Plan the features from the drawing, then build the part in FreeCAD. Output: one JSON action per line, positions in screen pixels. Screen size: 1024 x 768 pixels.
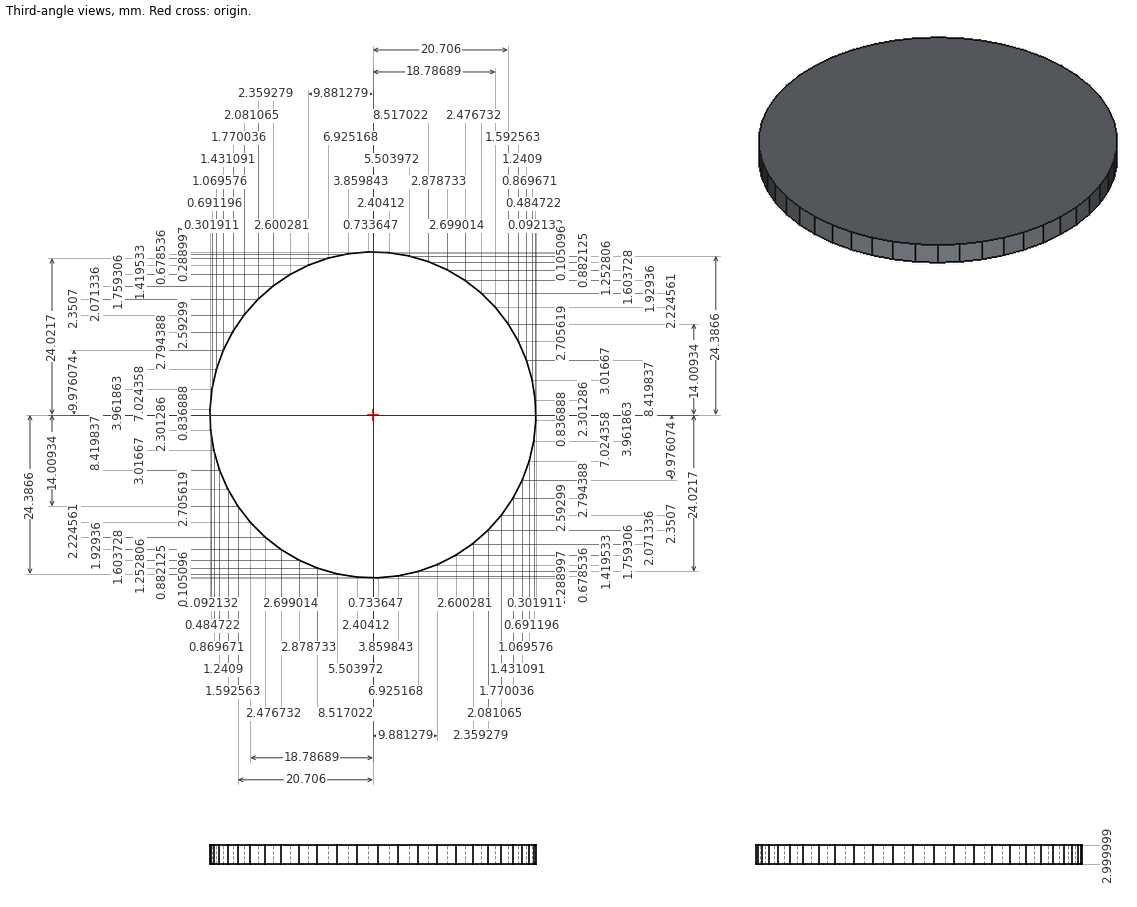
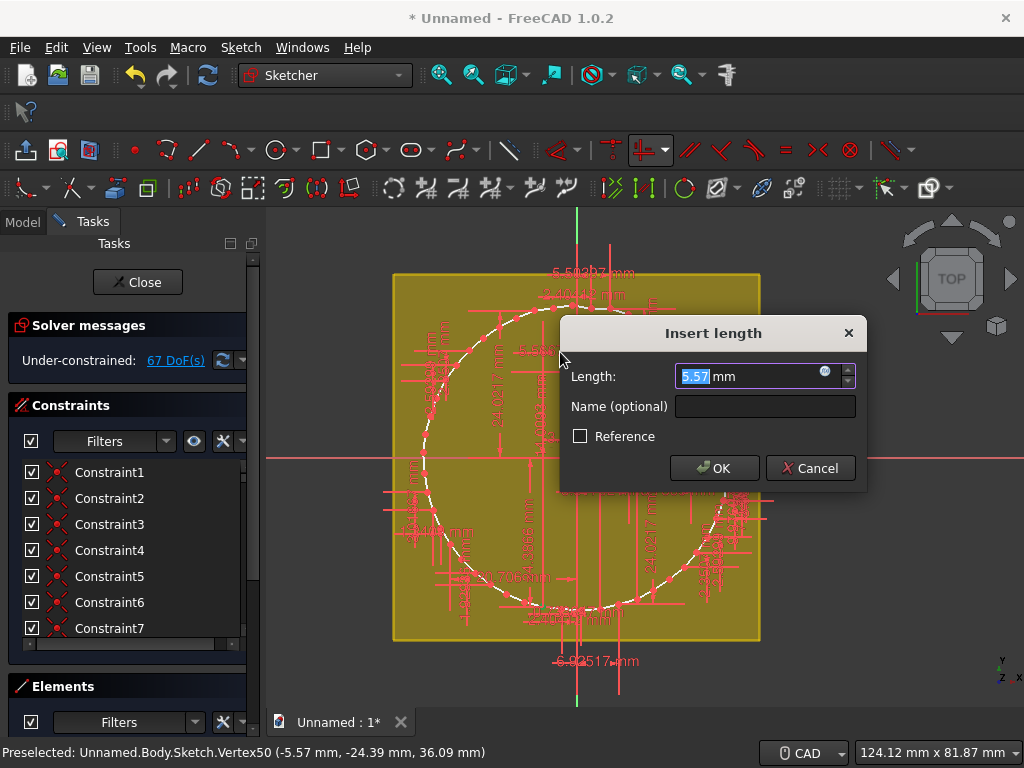
{"action": "type", "text": "5.503972"}
{"action": "key", "text": "Return"}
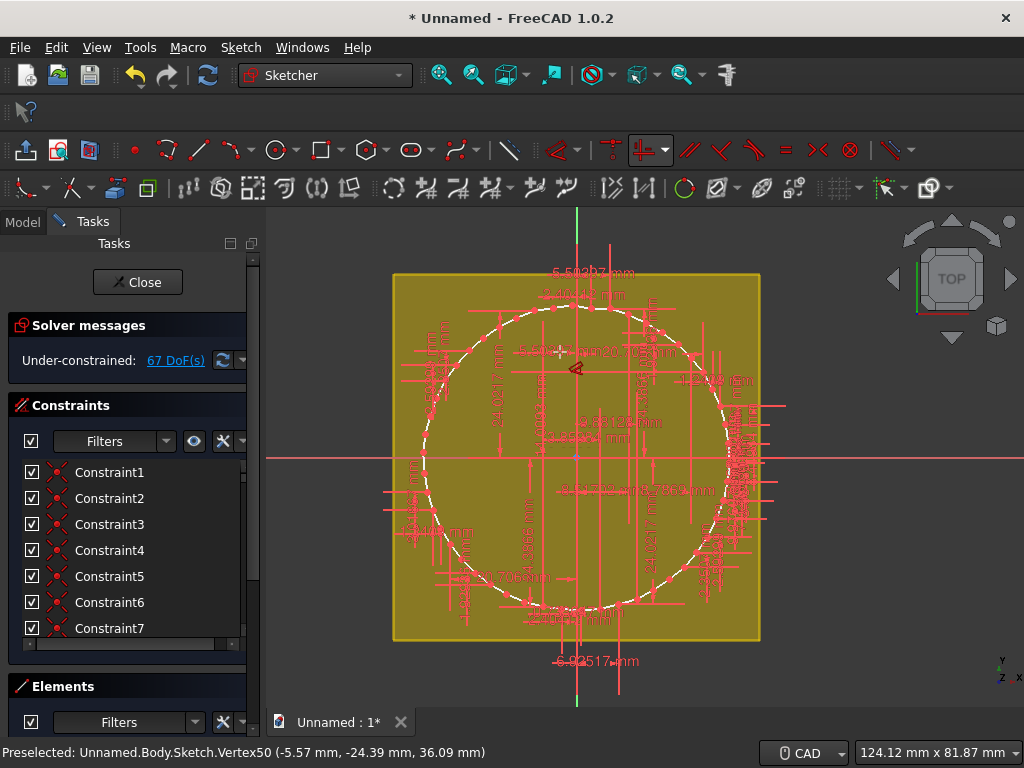
{"action": "left_click", "coordinate": [525, 602]}
{"action": "left_click", "coordinate": [551, 328]}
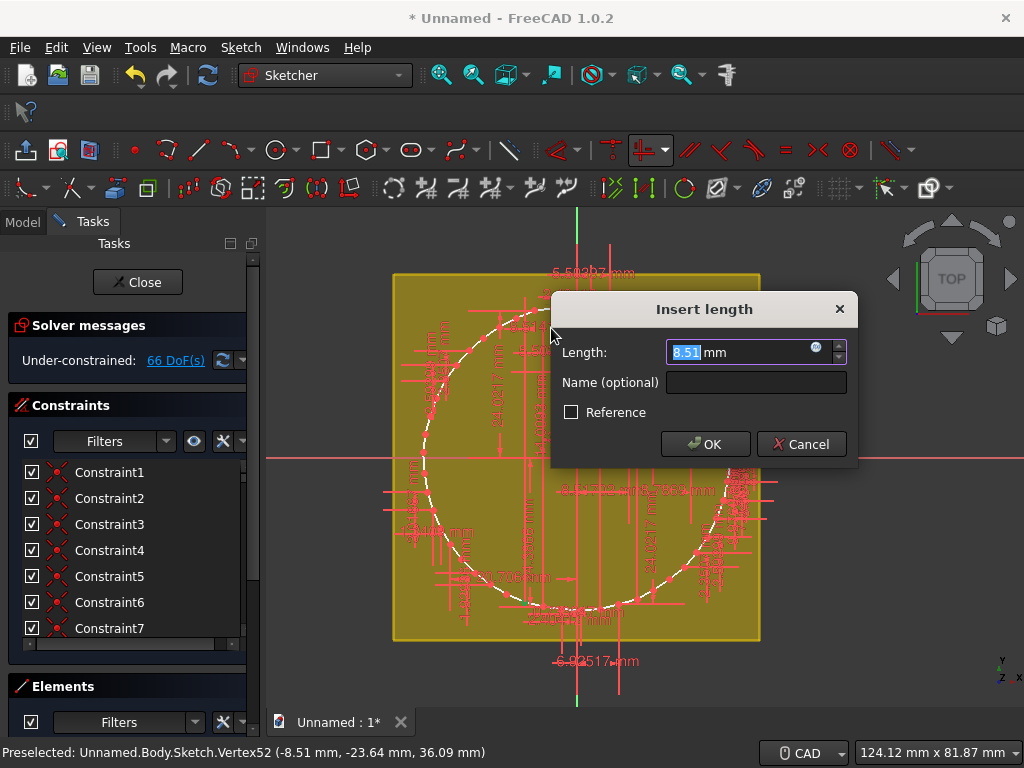
{"action": "type", "text": "8.517022"}
{"action": "key", "text": "Return"}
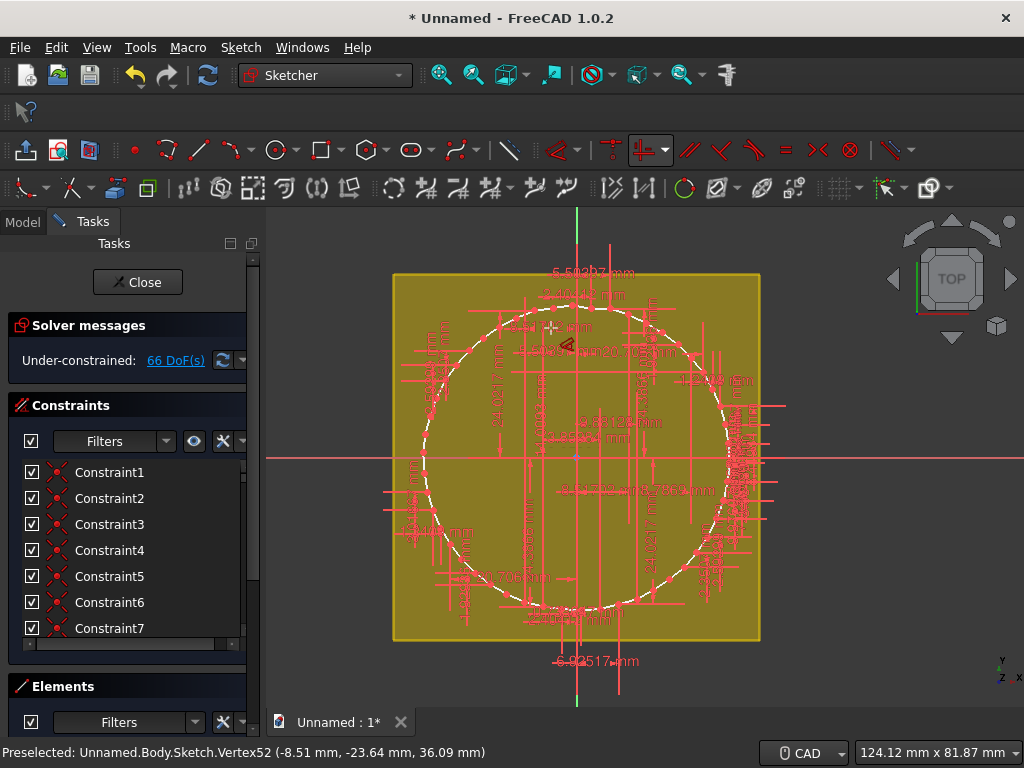
{"action": "left_click", "coordinate": [462, 559]}
{"action": "left_click", "coordinate": [493, 617]}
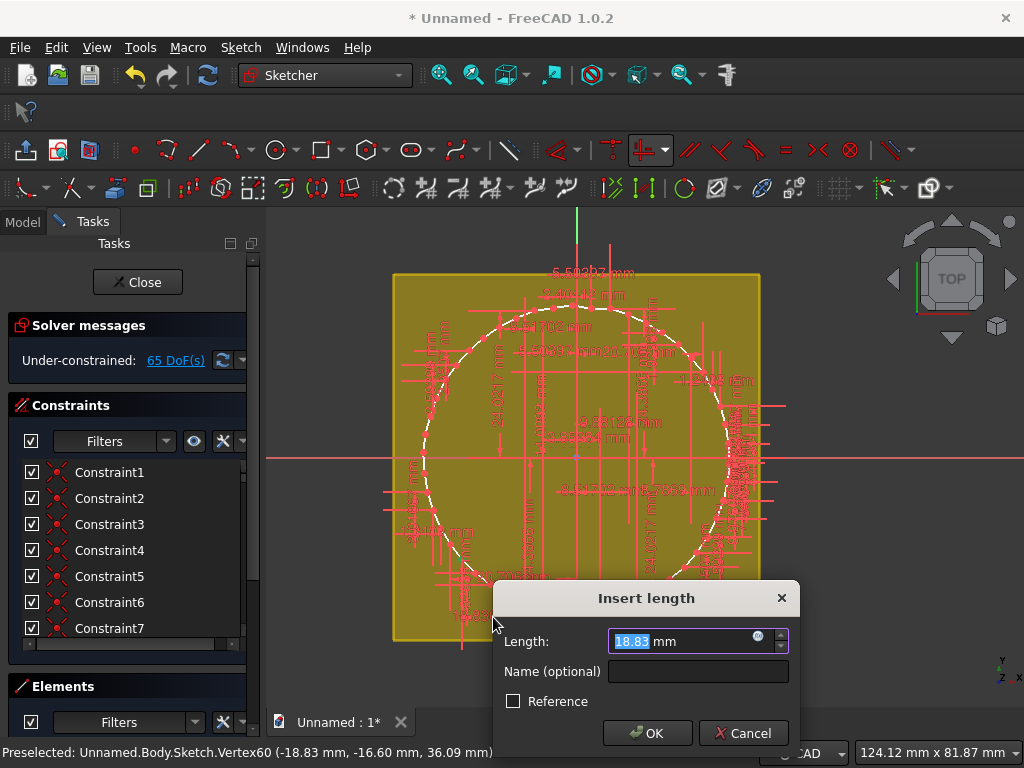
{"action": "type", "text": "18.78689"}
{"action": "key", "text": "Return"}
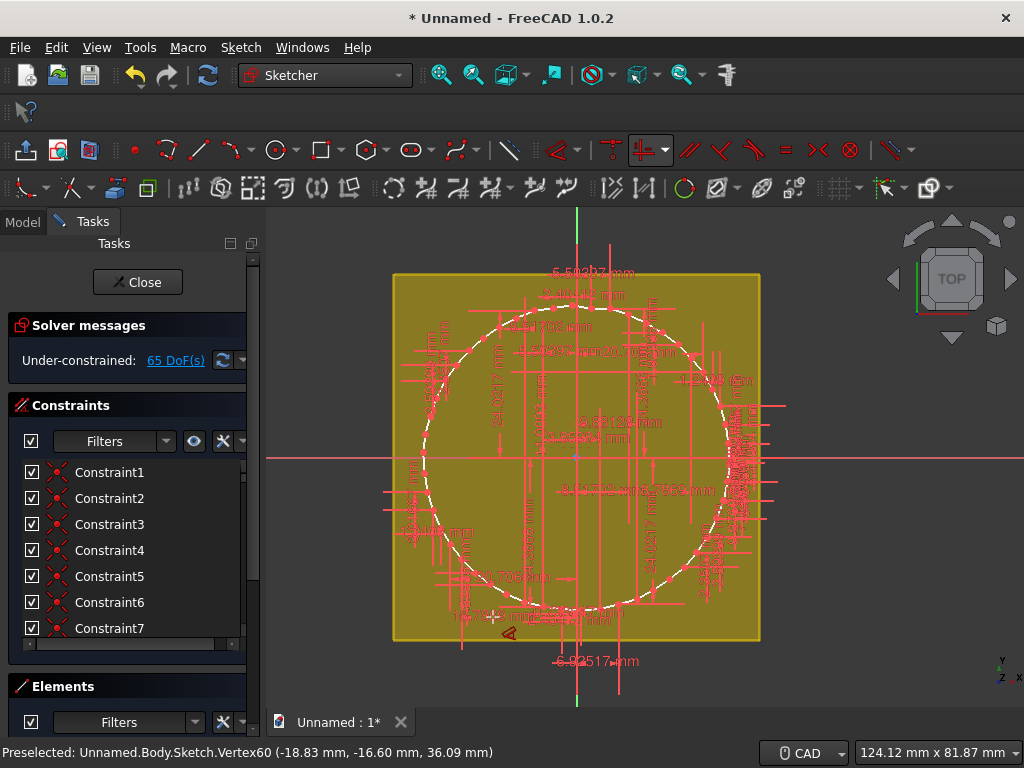
{"action": "left_click", "coordinate": [450, 544]}
{"action": "left_click", "coordinate": [392, 481]}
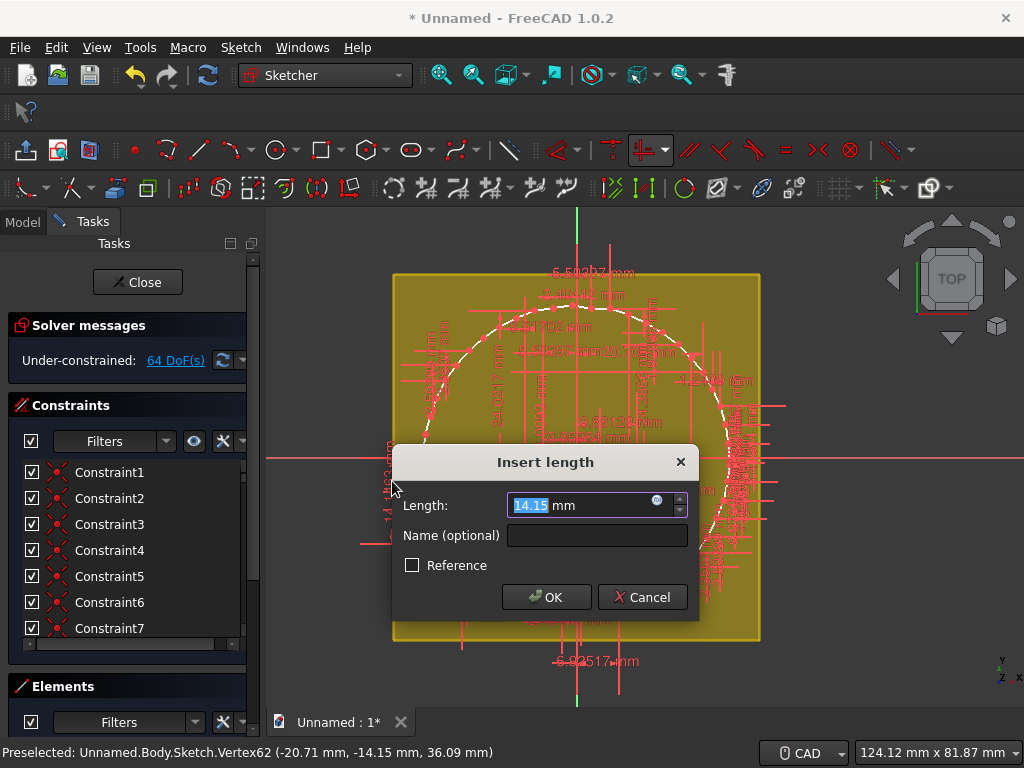
{"action": "type", "text": "14.00934"}
{"action": "key", "text": "Return"}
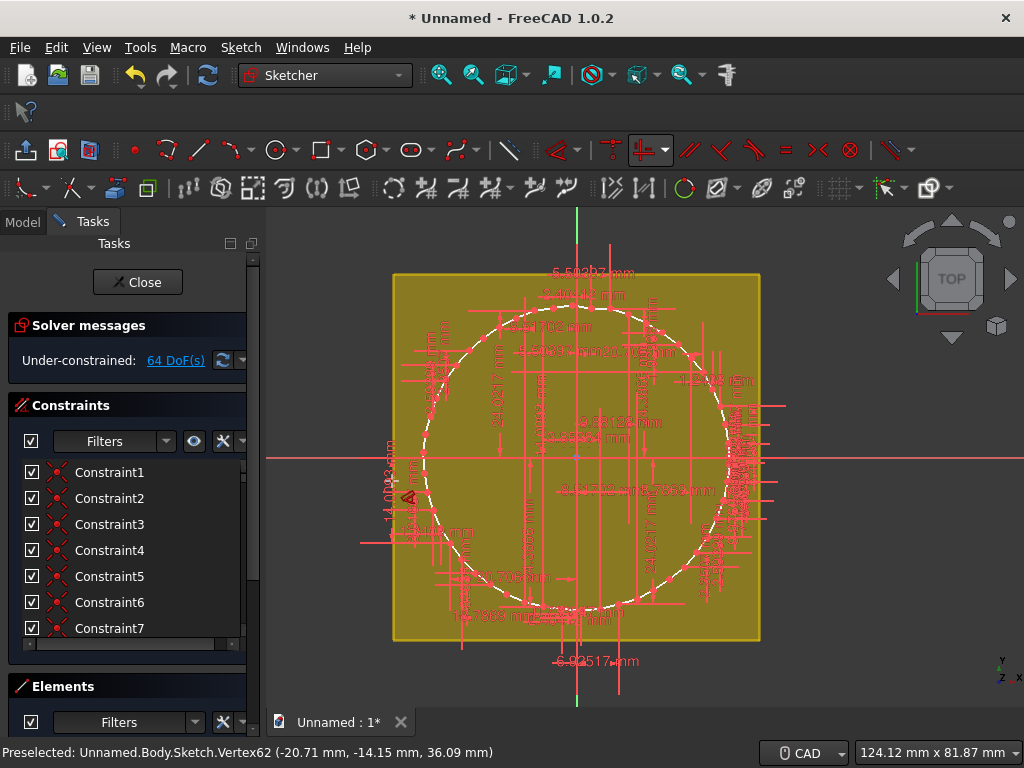
{"action": "left_click", "coordinate": [433, 510]}
{"action": "left_click", "coordinate": [327, 503]}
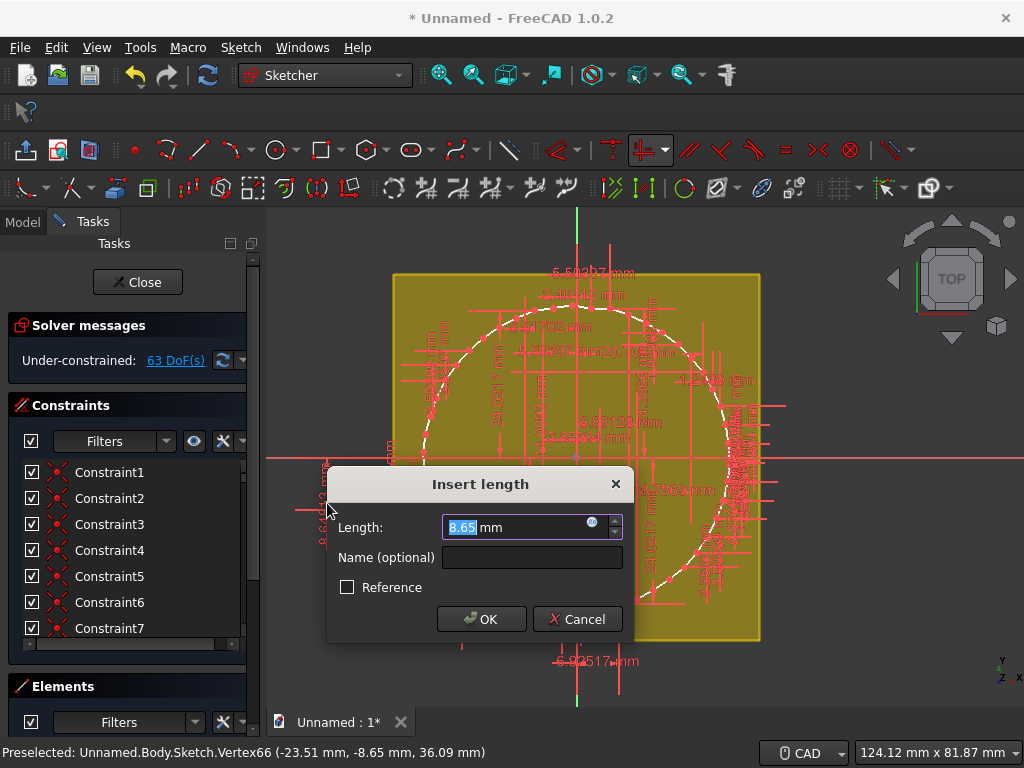
{"action": "type", "text": "8.419837"}
{"action": "key", "text": "Return"}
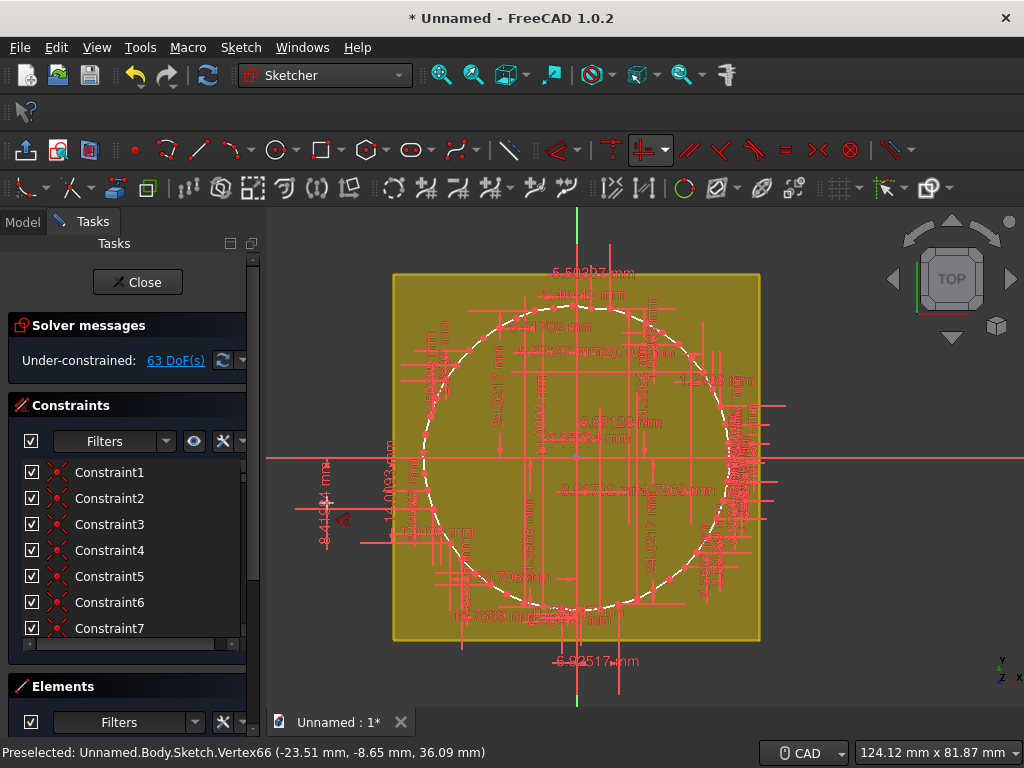
{"action": "scroll", "coordinate": [425, 473], "scroll_direction": "up", "scroll_amount": 6}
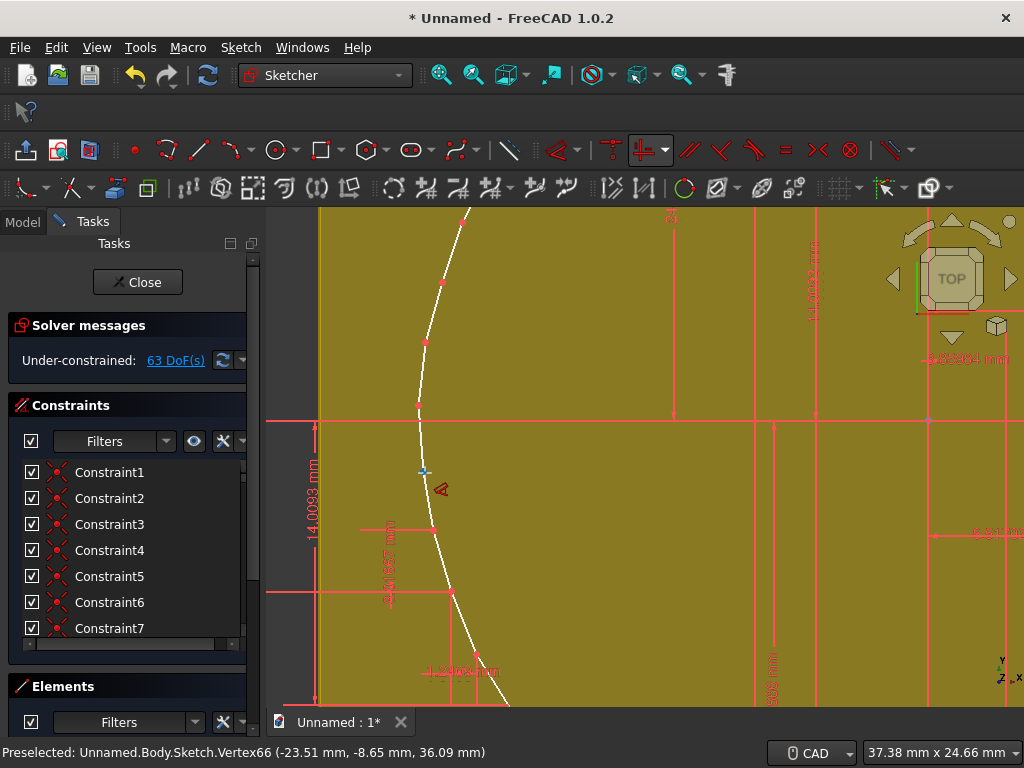
{"action": "left_click", "coordinate": [423, 472]}
{"action": "left_click", "coordinate": [389, 446]}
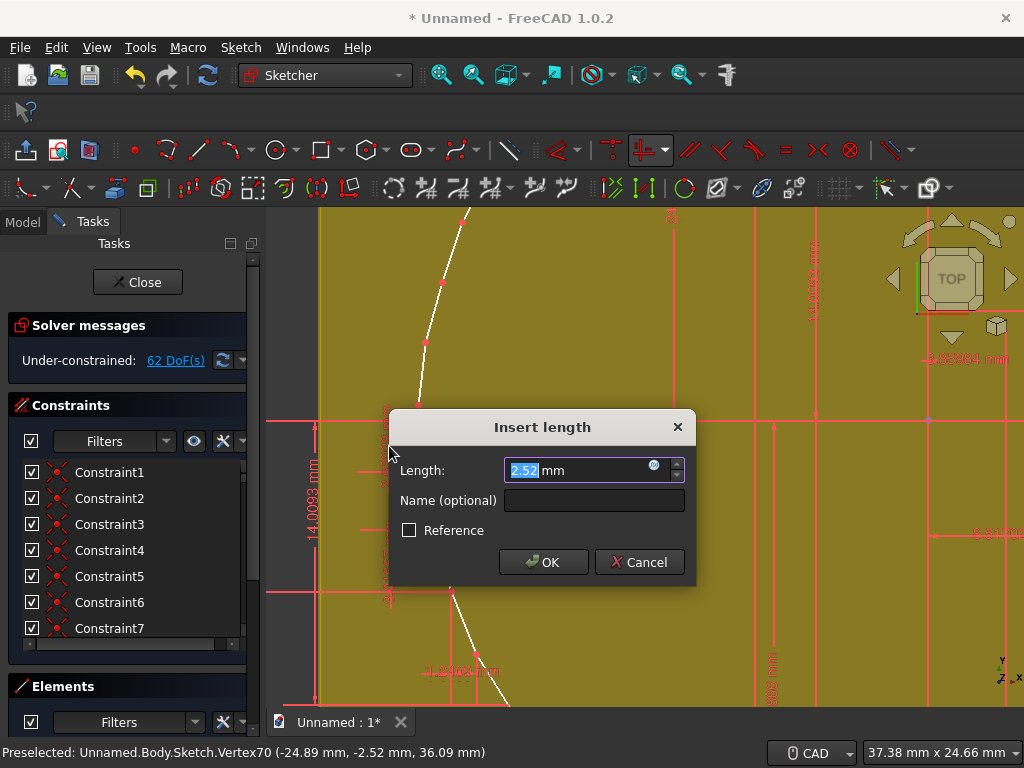
{"action": "type", "text": "2.301286"}
{"action": "key", "text": "Return"}